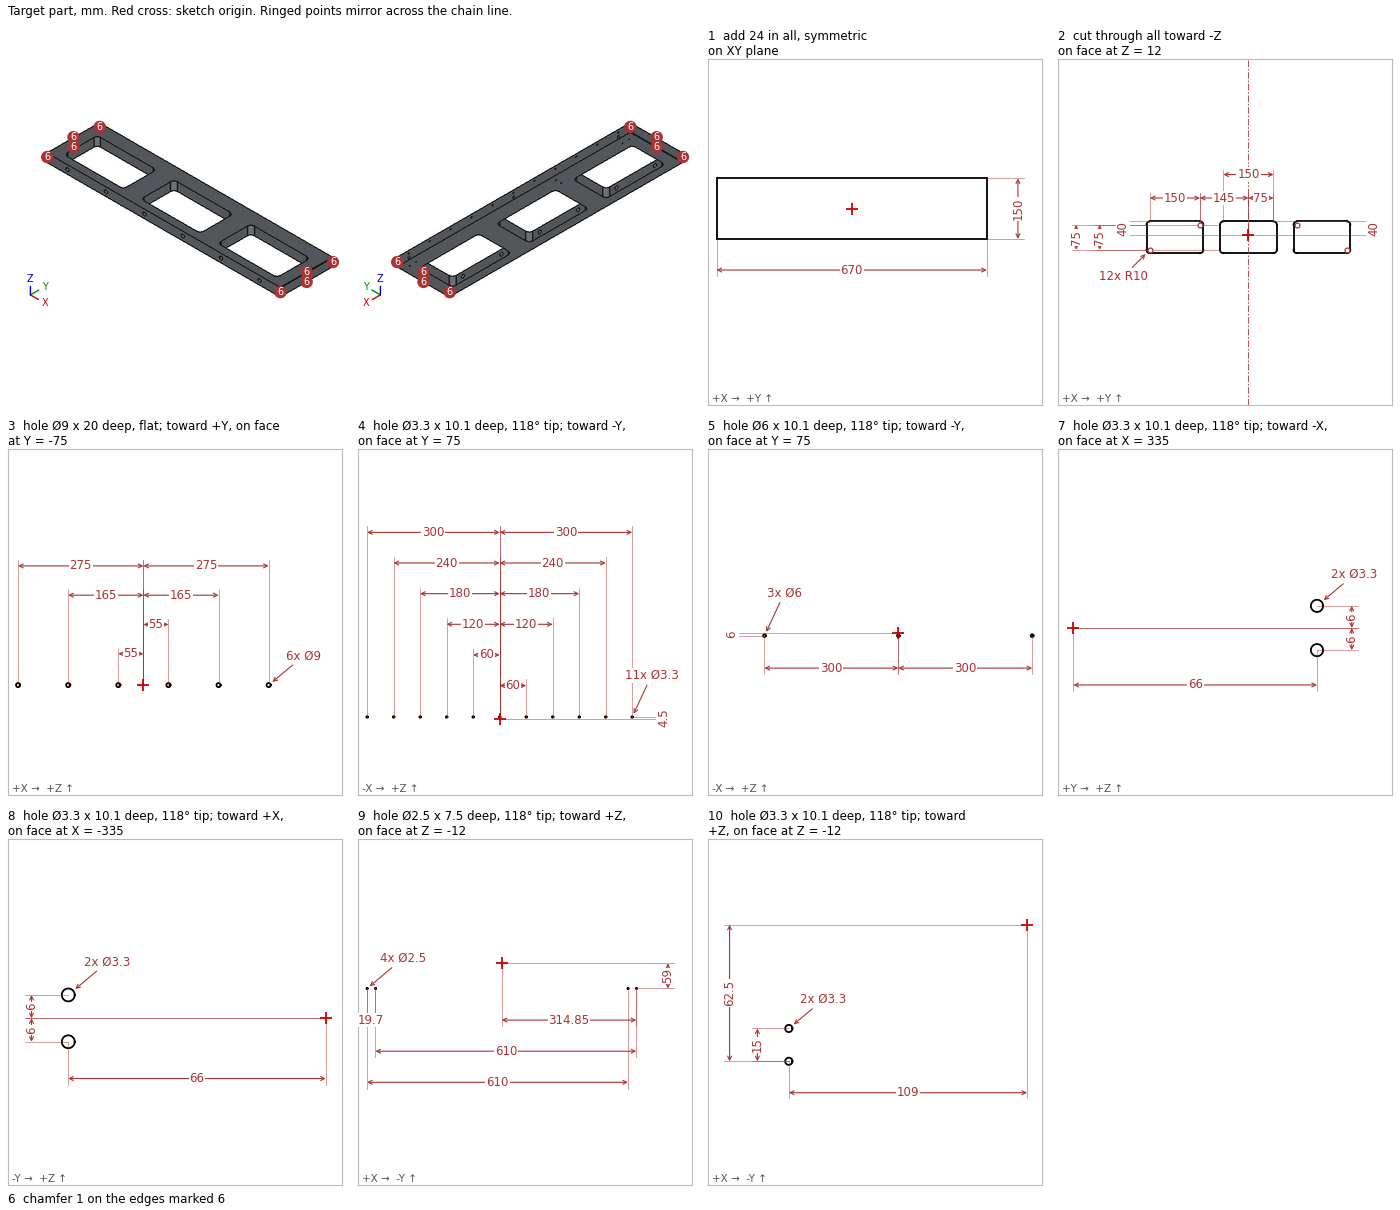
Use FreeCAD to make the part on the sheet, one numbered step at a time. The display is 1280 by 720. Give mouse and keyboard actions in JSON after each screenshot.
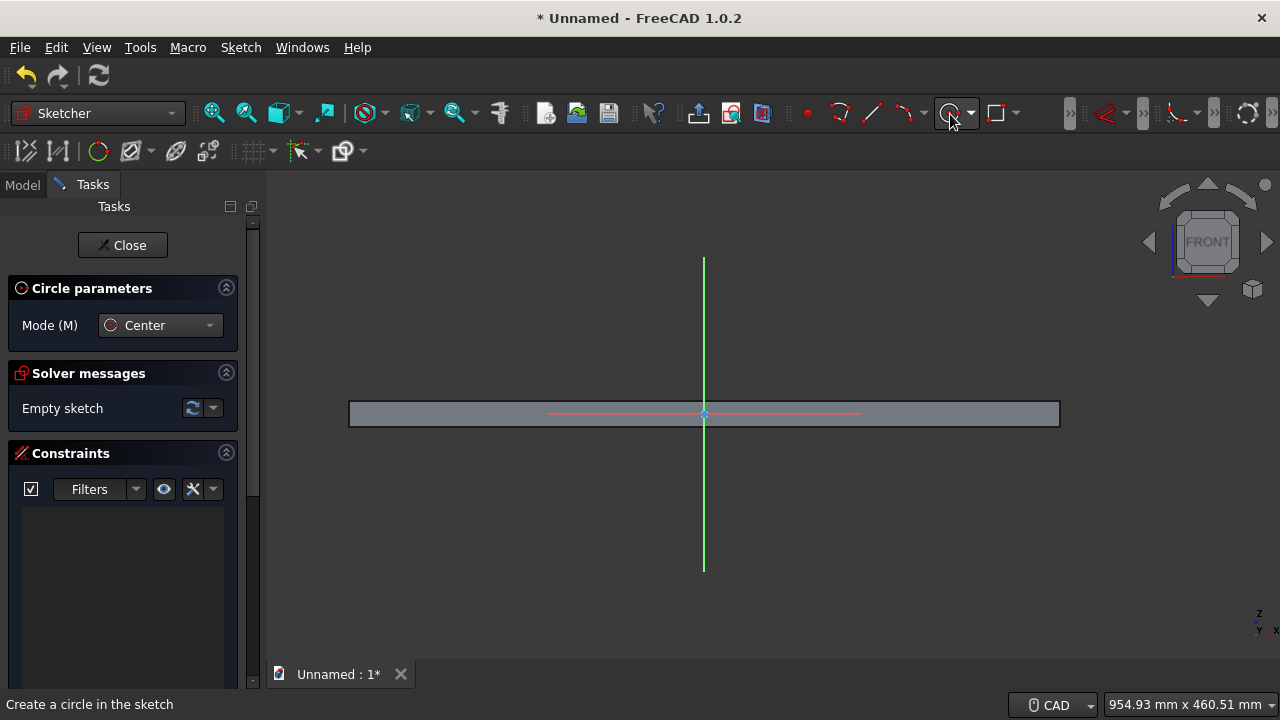
{"action": "scroll", "coordinate": [996, 414], "scroll_direction": "up", "scroll_amount": 8}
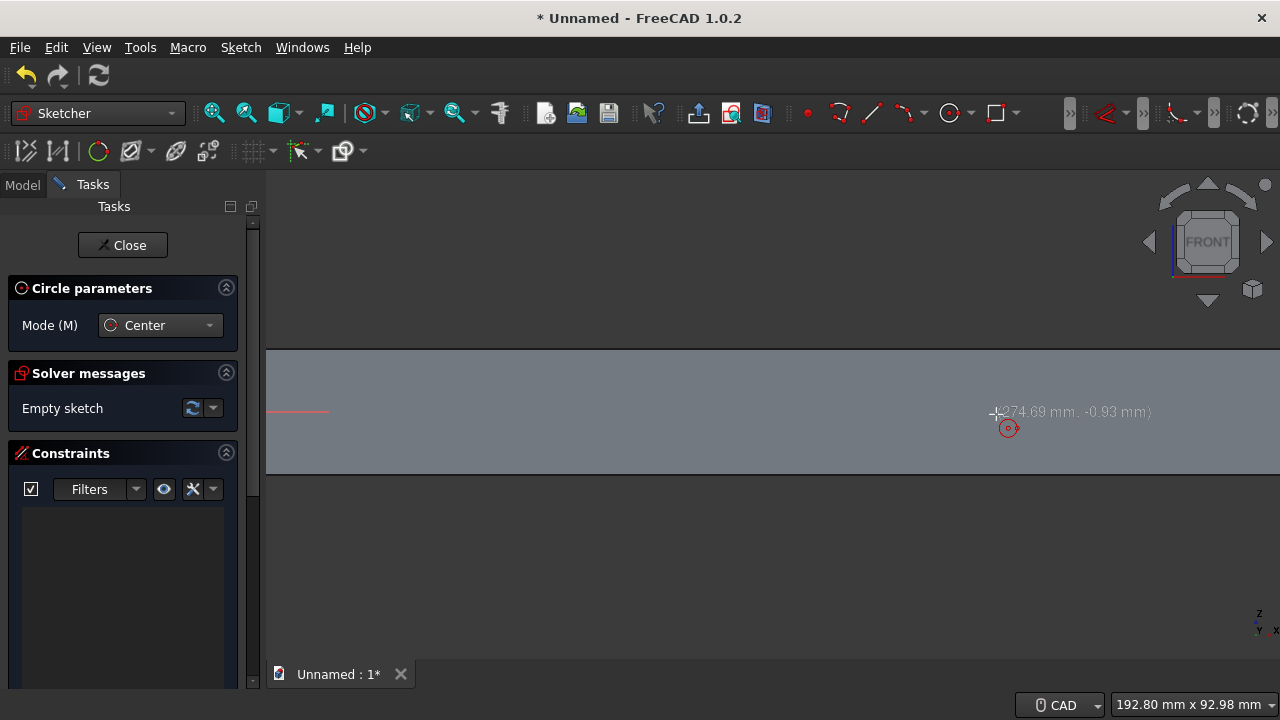
{"action": "scroll", "coordinate": [997, 415], "scroll_direction": "down", "scroll_amount": 8}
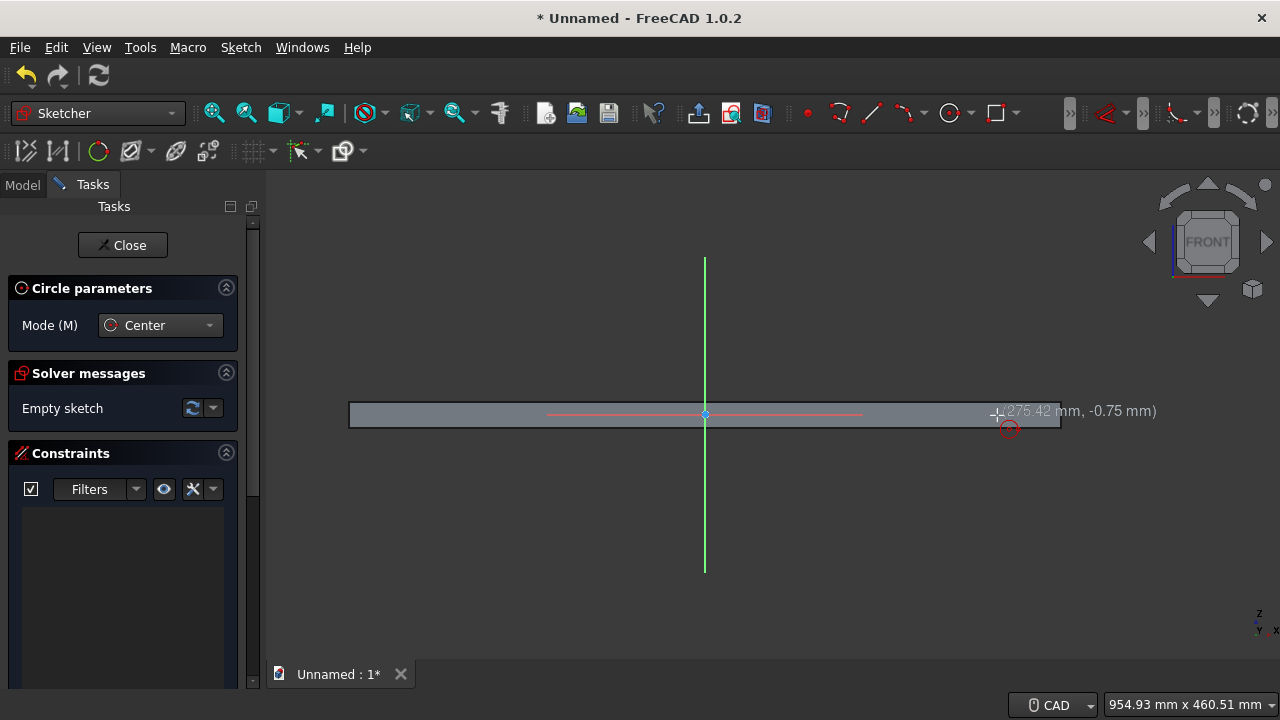
{"action": "left_click", "coordinate": [997, 415]}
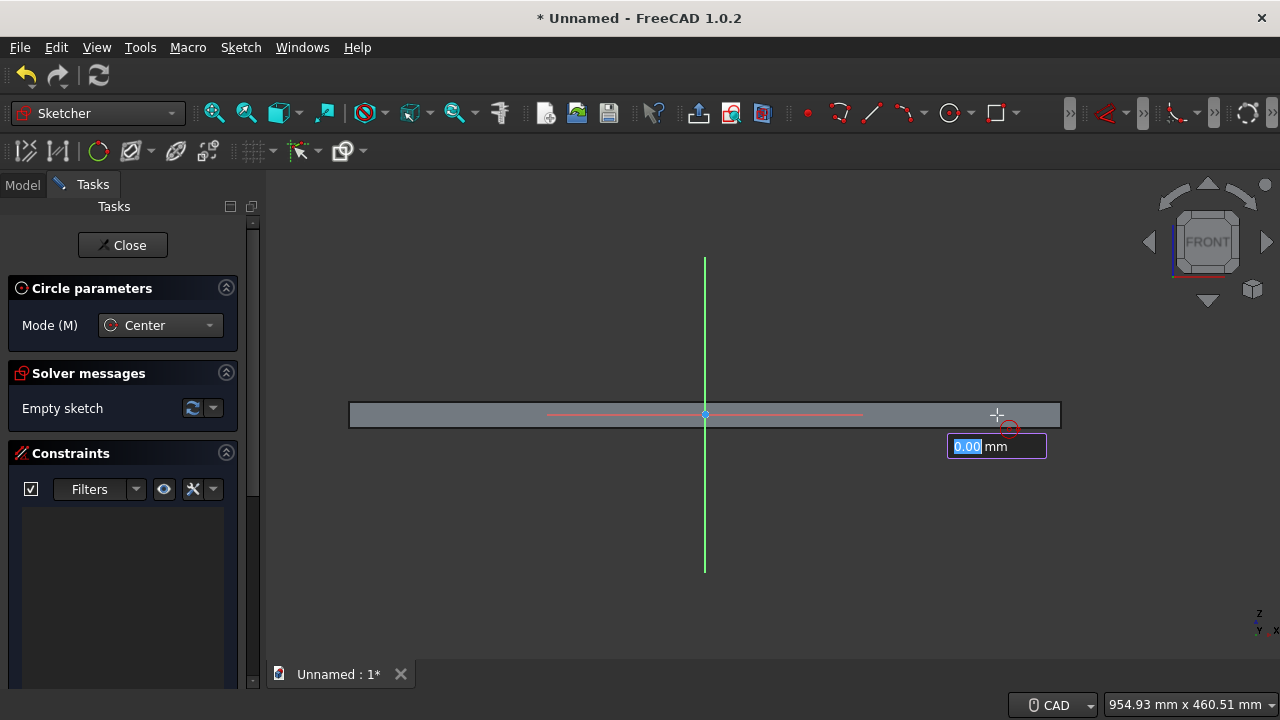
{"action": "scroll", "coordinate": [995, 419], "scroll_direction": "up", "scroll_amount": 7}
{"action": "mouse_move", "coordinate": [995, 419]}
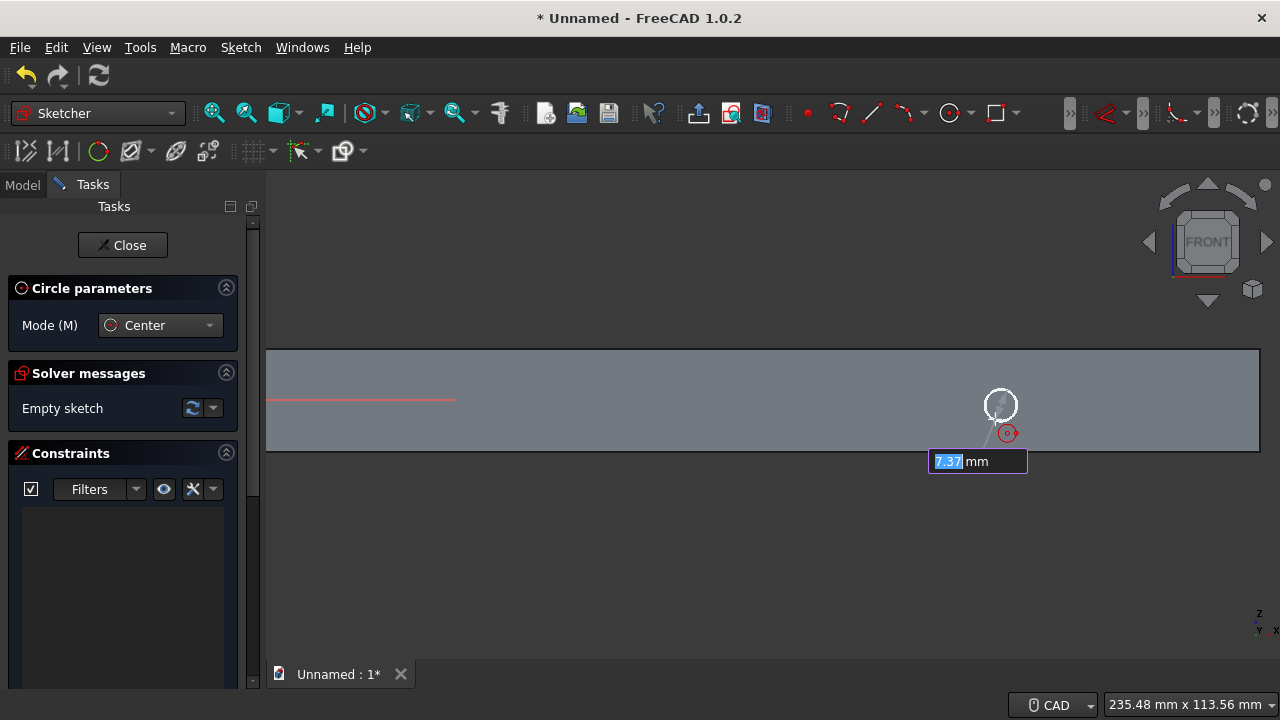
{"action": "type", "text": "9"}
{"action": "key", "text": "Return"}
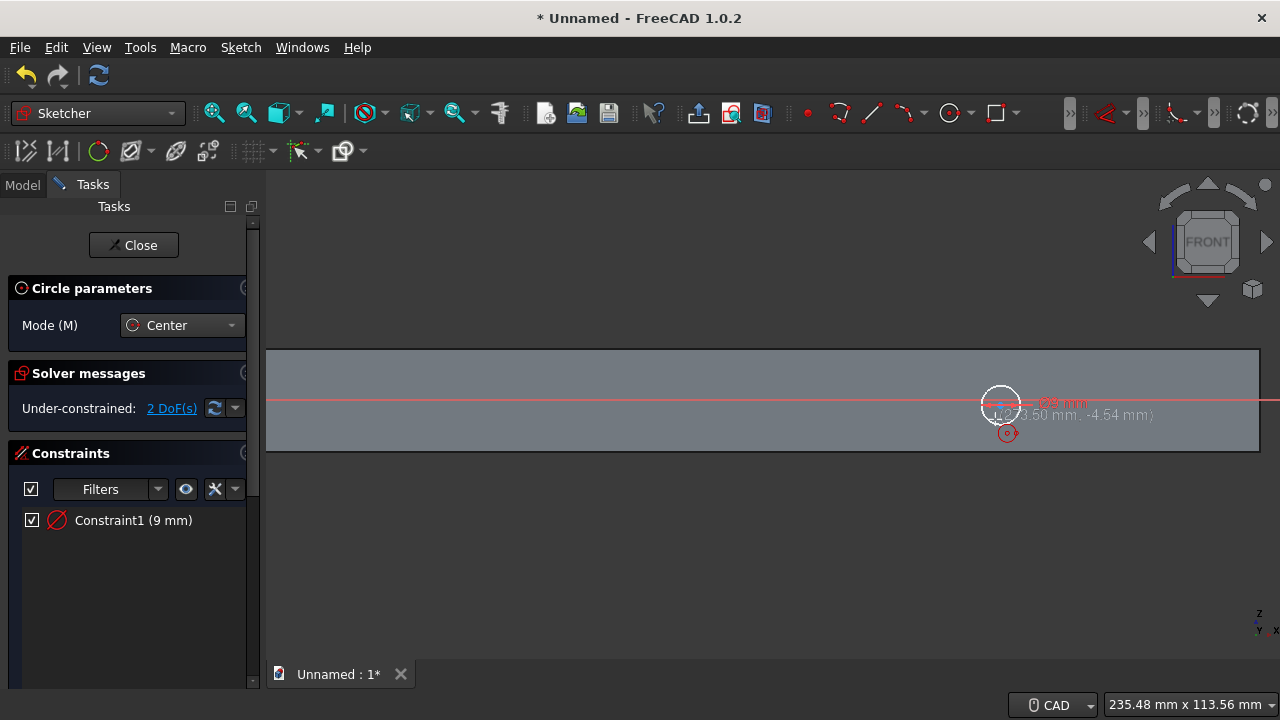
{"action": "scroll", "coordinate": [995, 419], "scroll_direction": "down", "scroll_amount": 7}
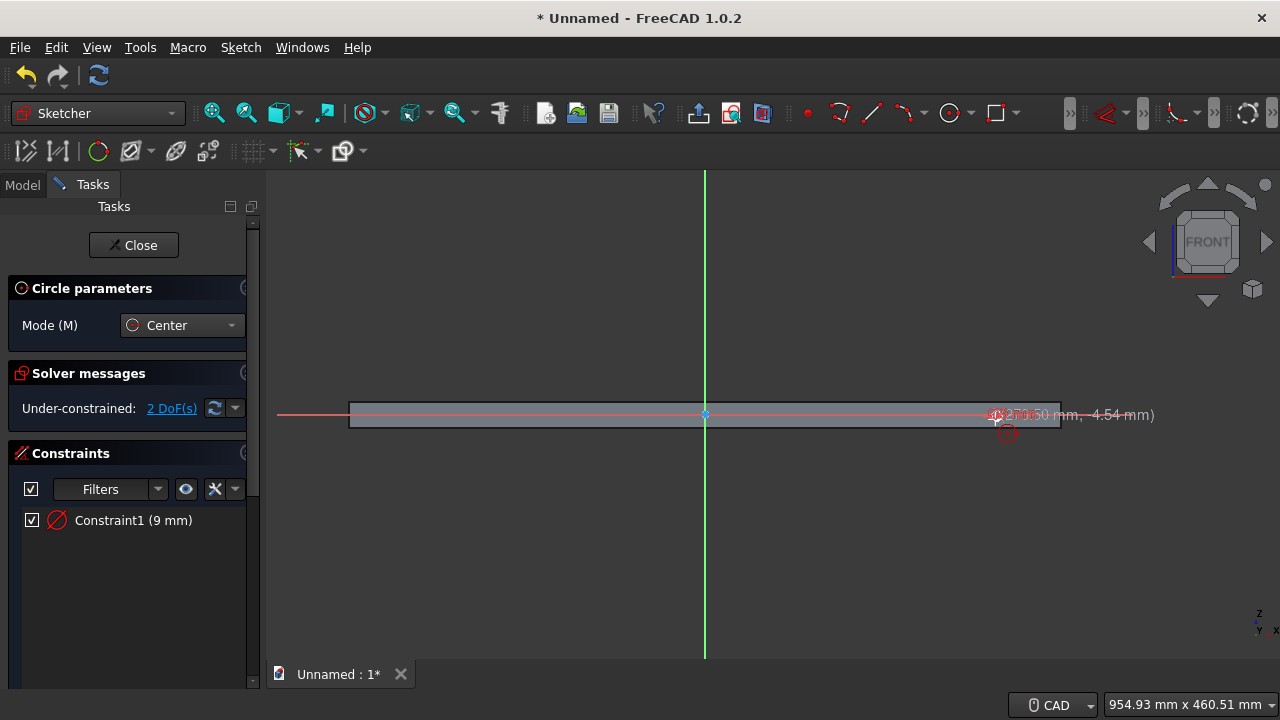
{"action": "scroll", "coordinate": [413, 415], "scroll_direction": "up", "scroll_amount": 8}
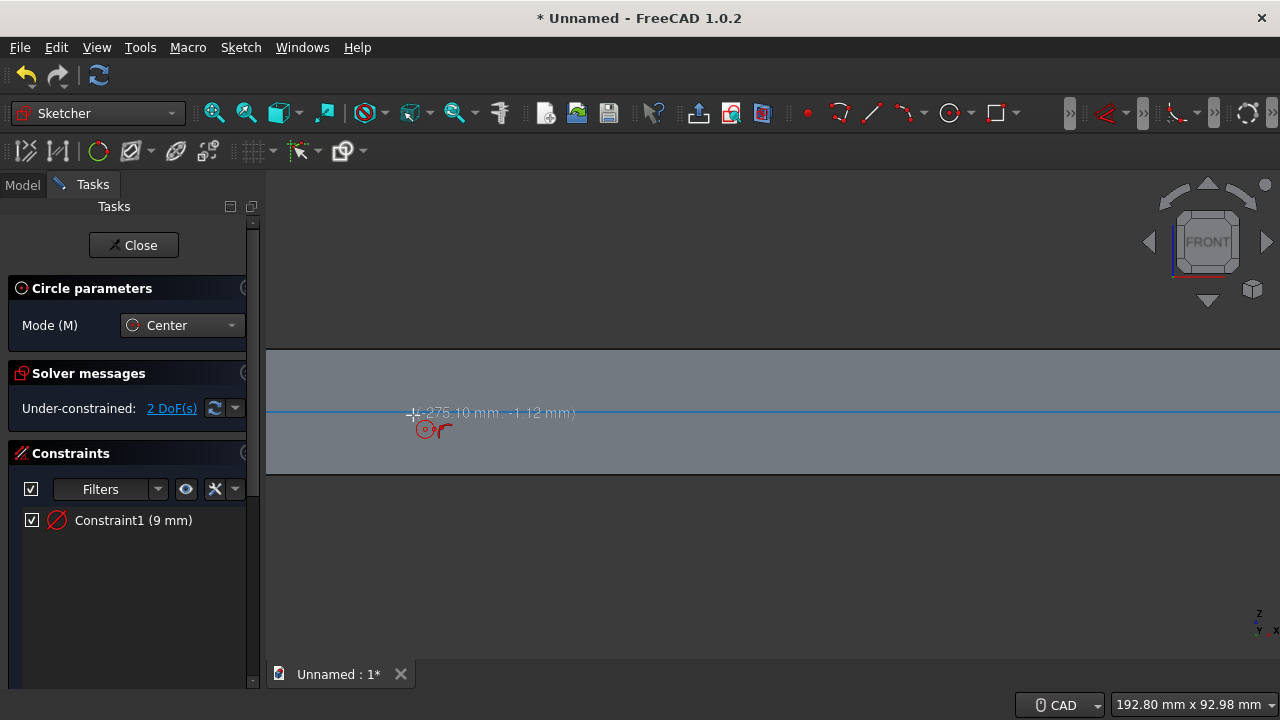
{"action": "scroll", "coordinate": [412, 415], "scroll_direction": "down", "scroll_amount": 8}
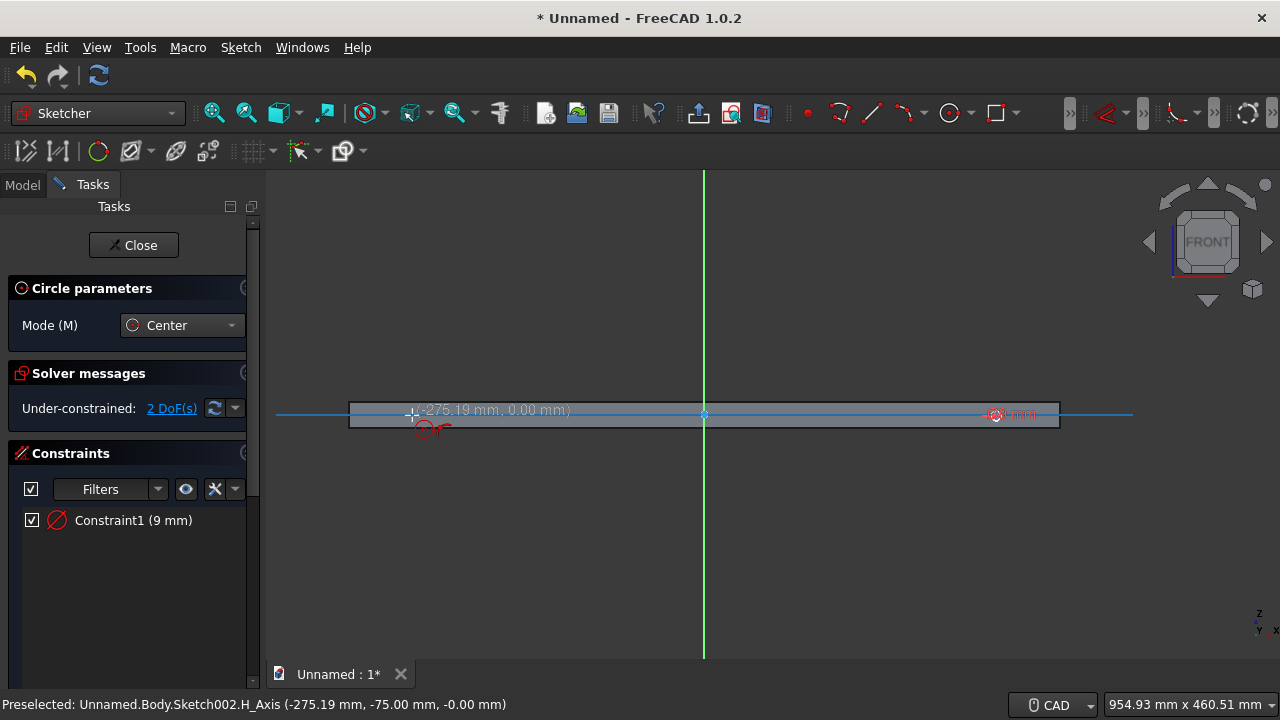
{"action": "left_click", "coordinate": [412, 415]}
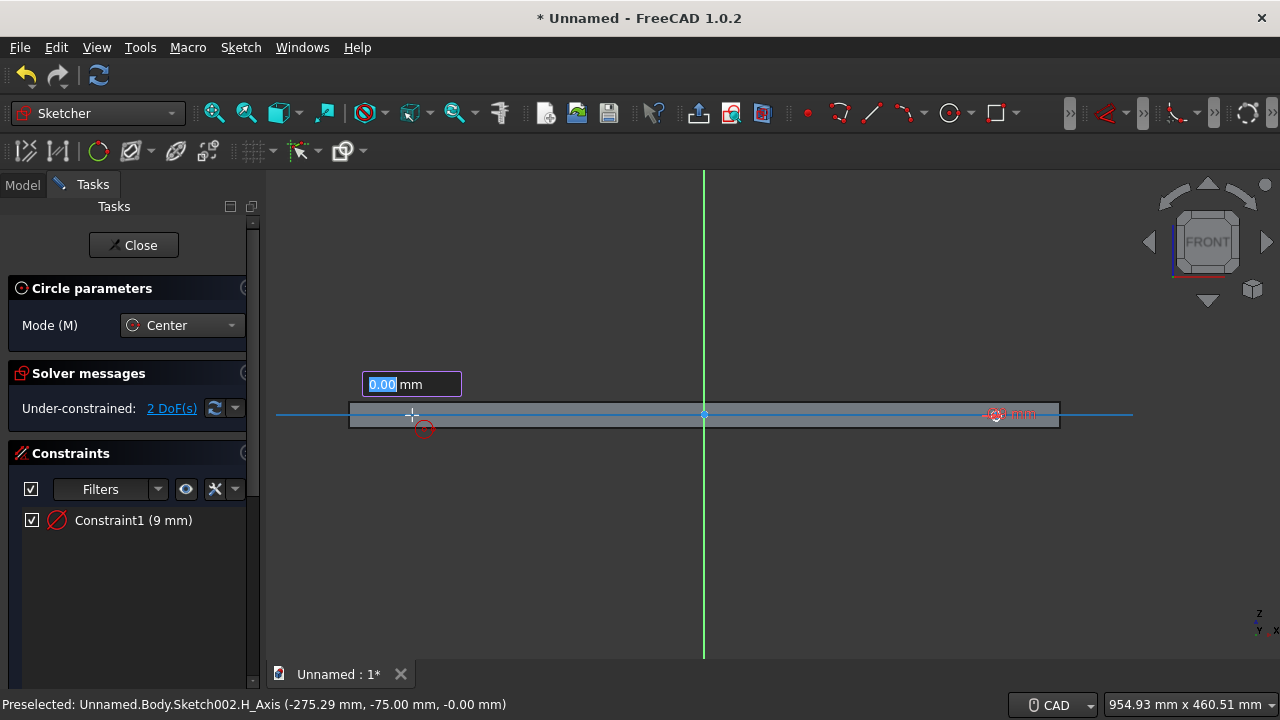
{"action": "scroll", "coordinate": [411, 419], "scroll_direction": "up", "scroll_amount": 7}
{"action": "mouse_move", "coordinate": [409, 419]}